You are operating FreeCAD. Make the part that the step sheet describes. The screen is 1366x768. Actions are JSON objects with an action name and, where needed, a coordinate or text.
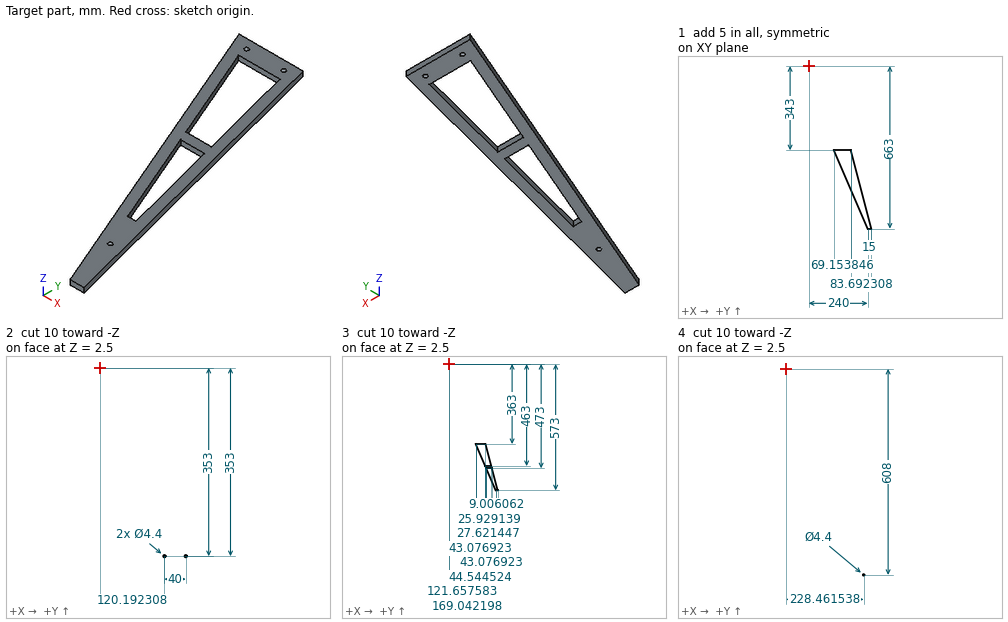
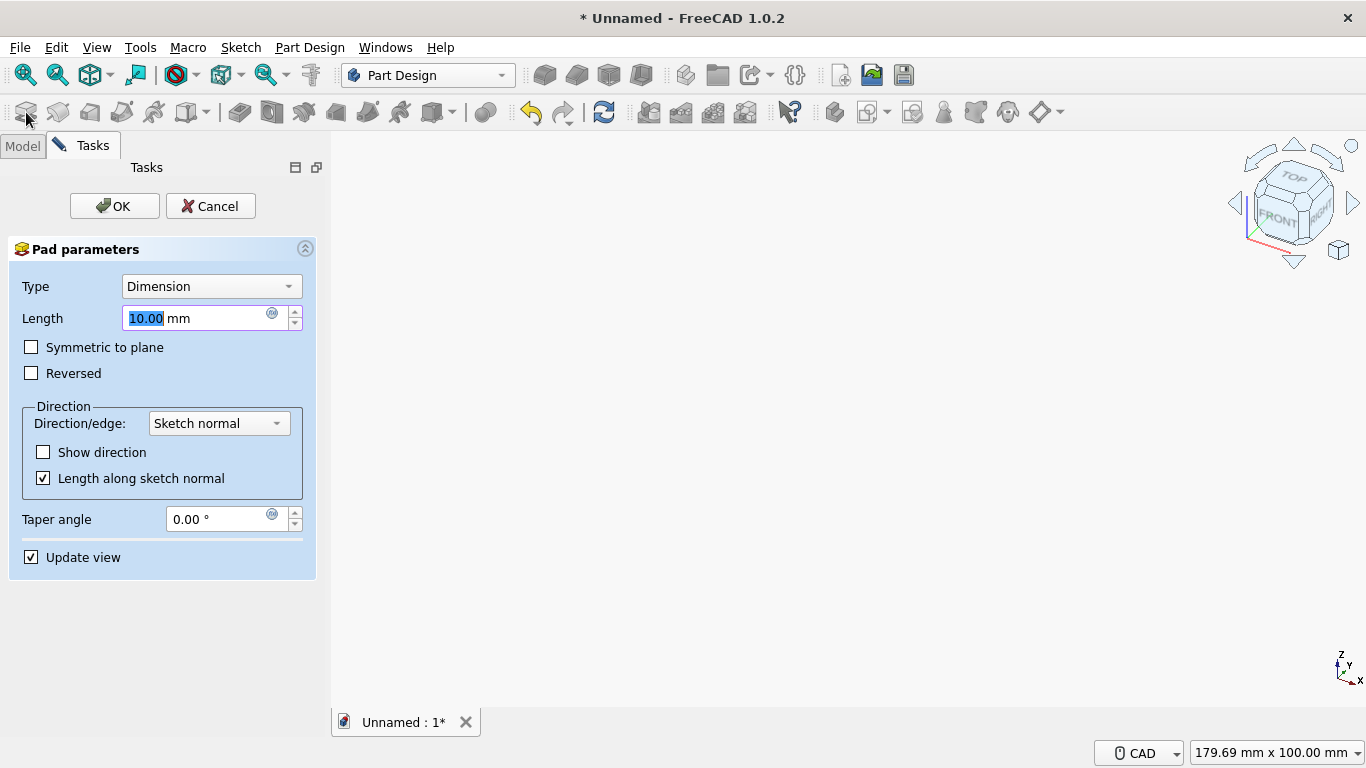
{"action": "type", "text": "5"}
{"action": "key", "text": "Tab"}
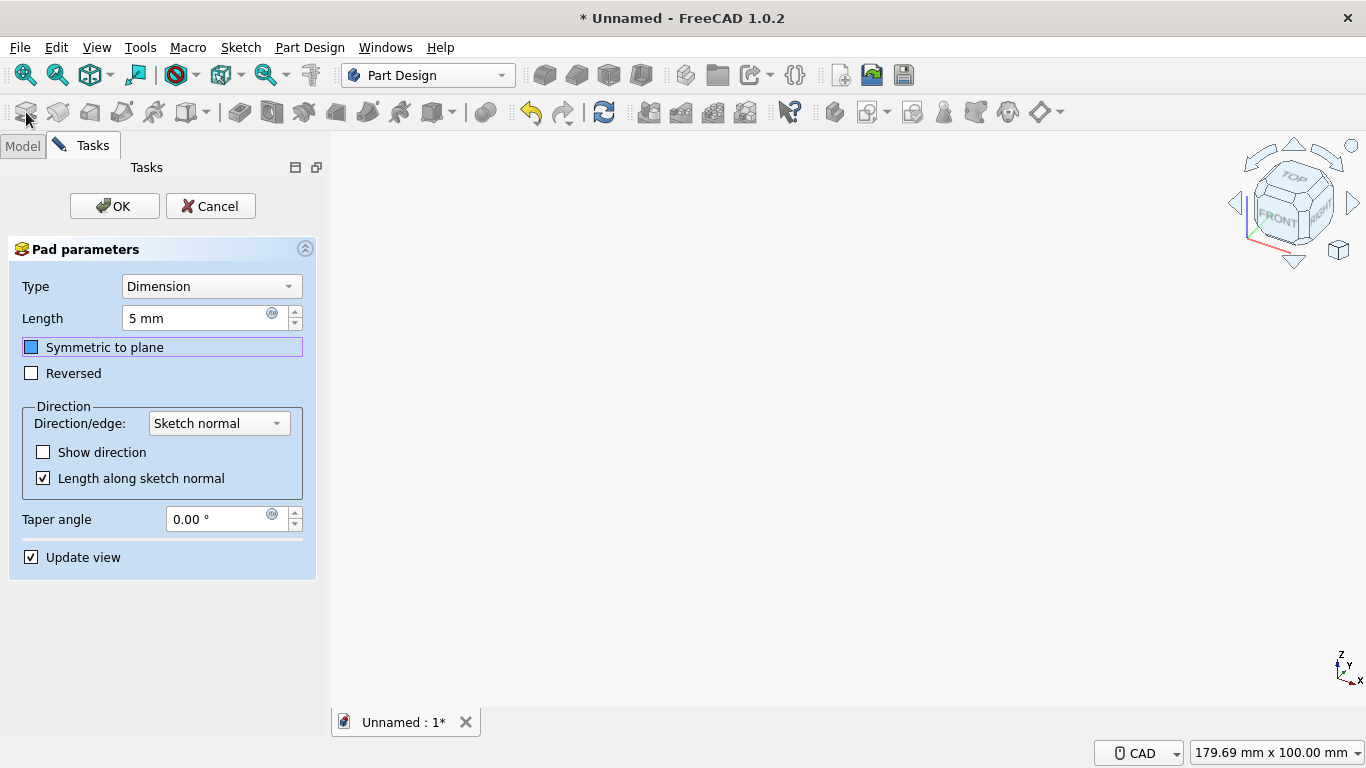
{"action": "left_click", "coordinate": [30, 347]}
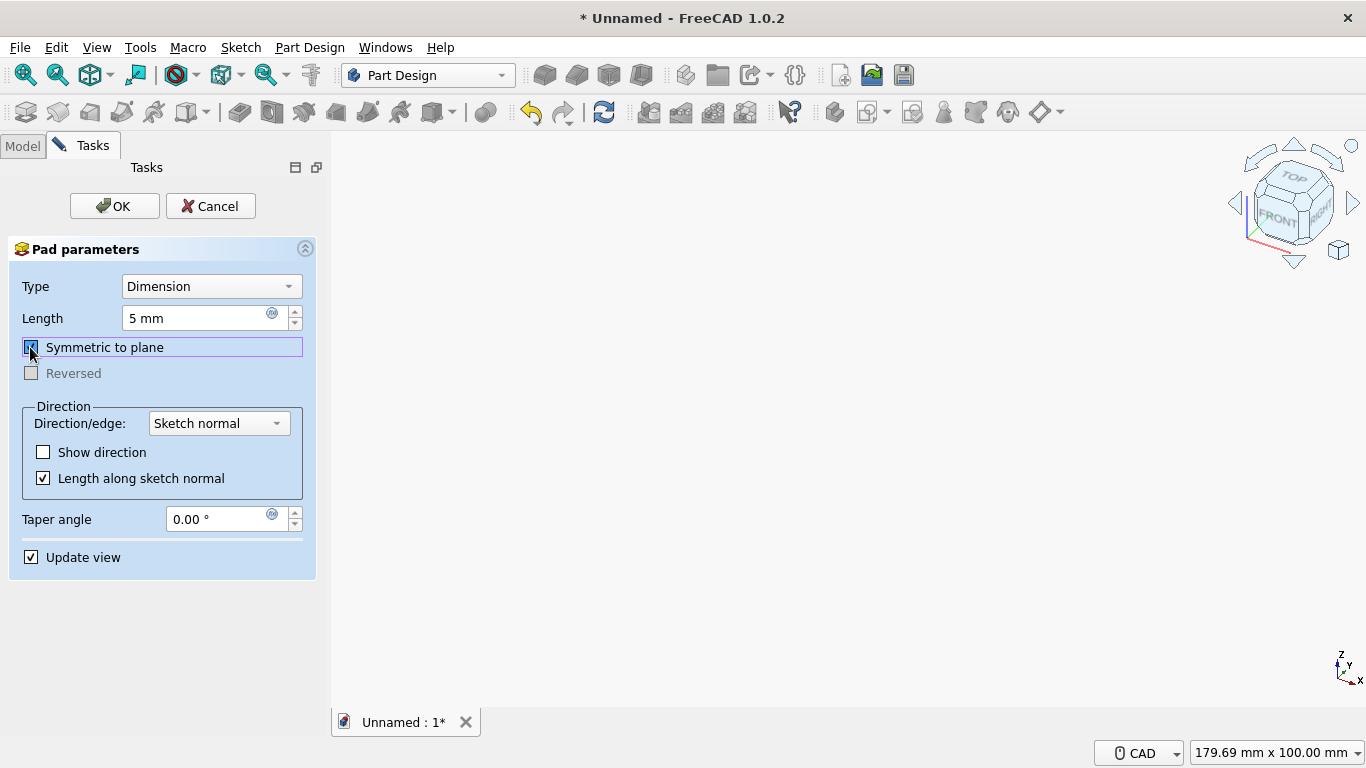
{"action": "left_click", "coordinate": [115, 206]}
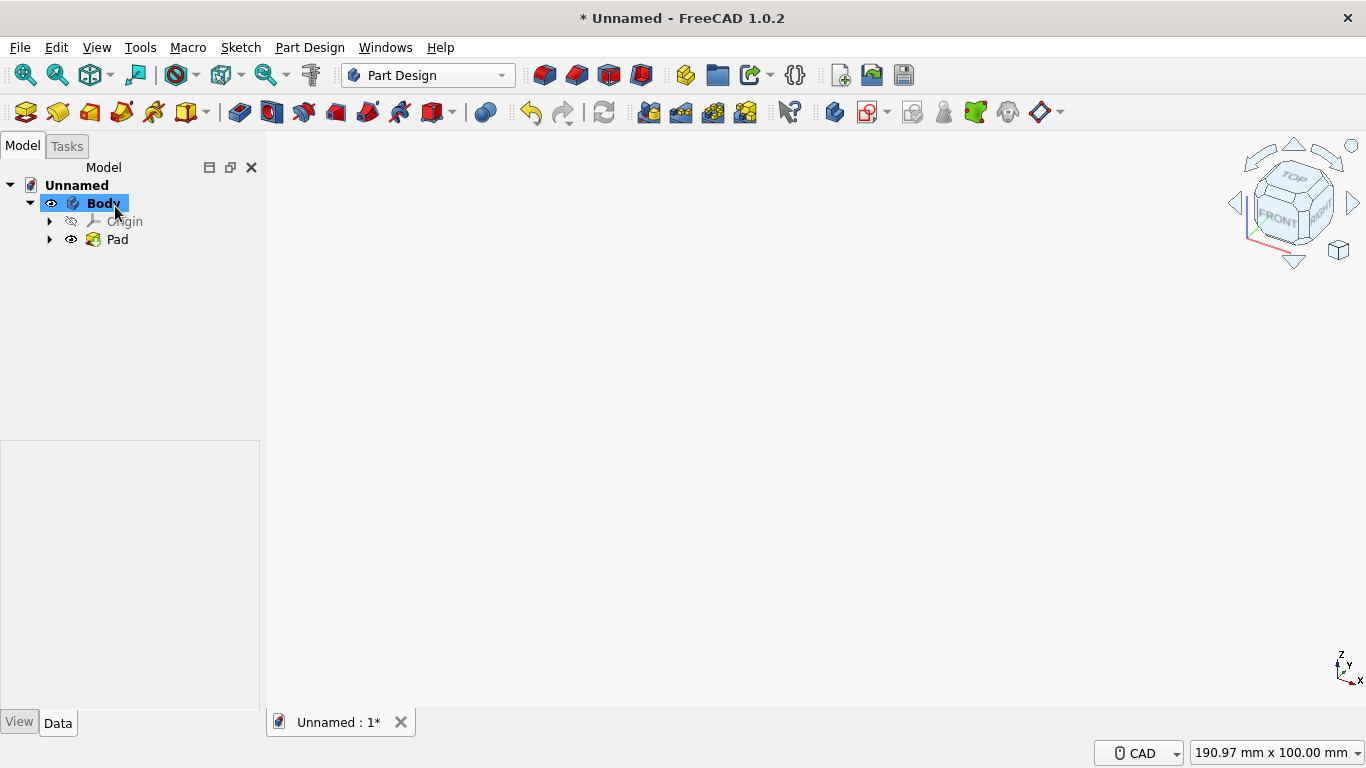
{"action": "key", "text": "v f"}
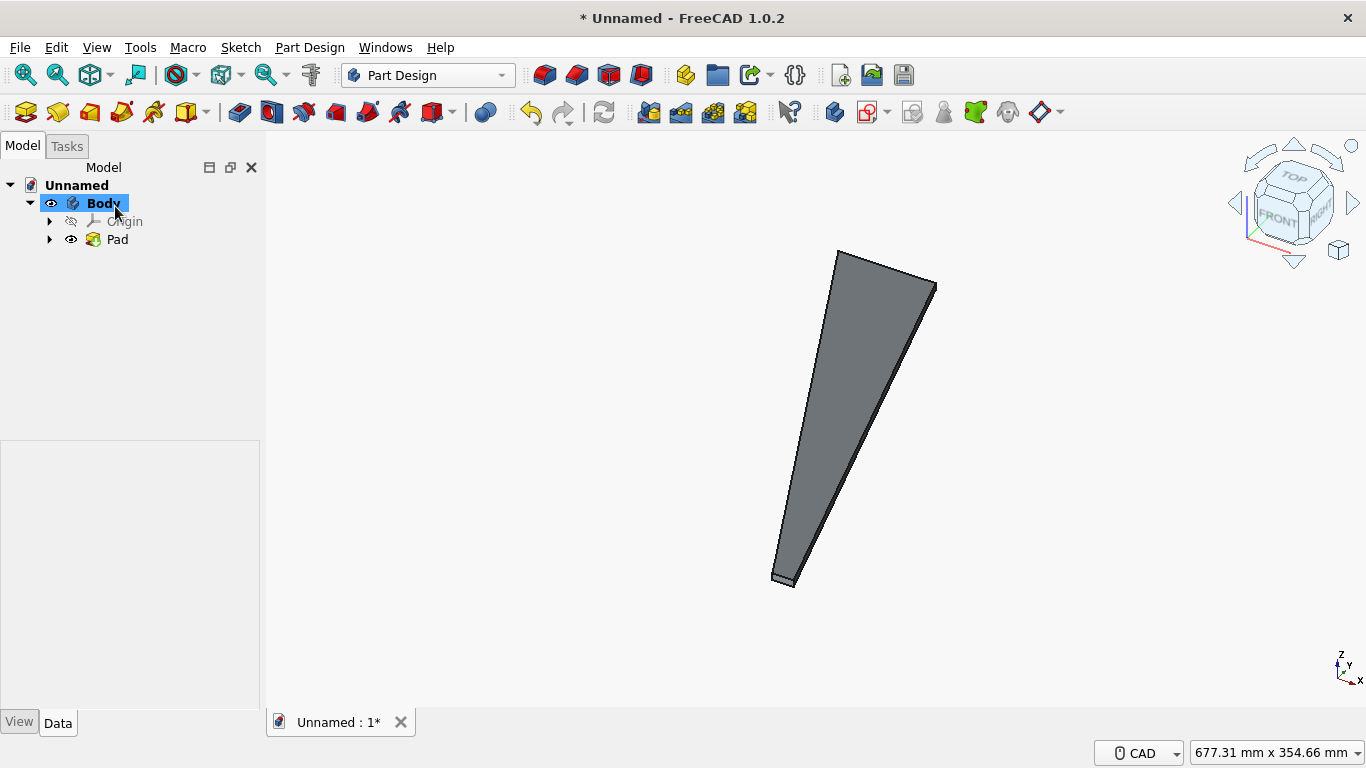
{"action": "left_click", "coordinate": [860, 331]}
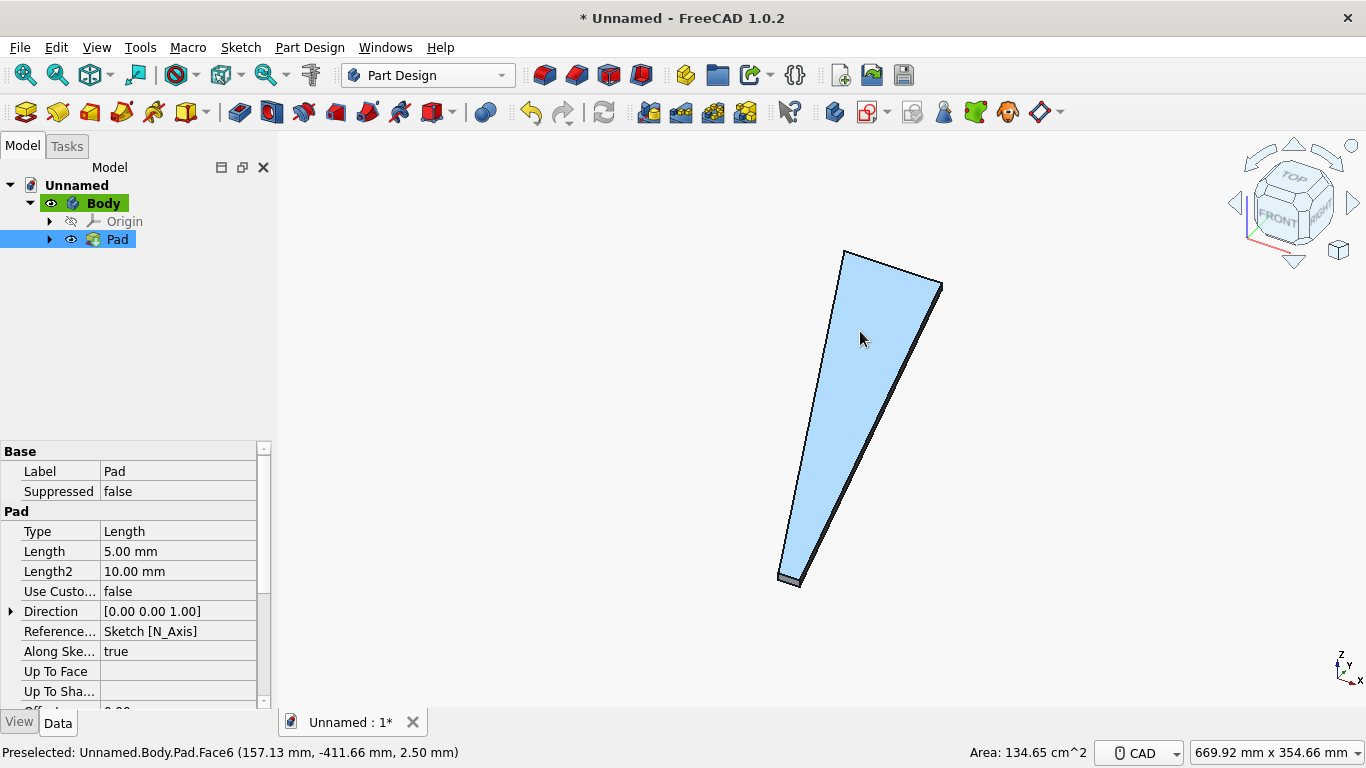
{"action": "left_click", "coordinate": [868, 112]}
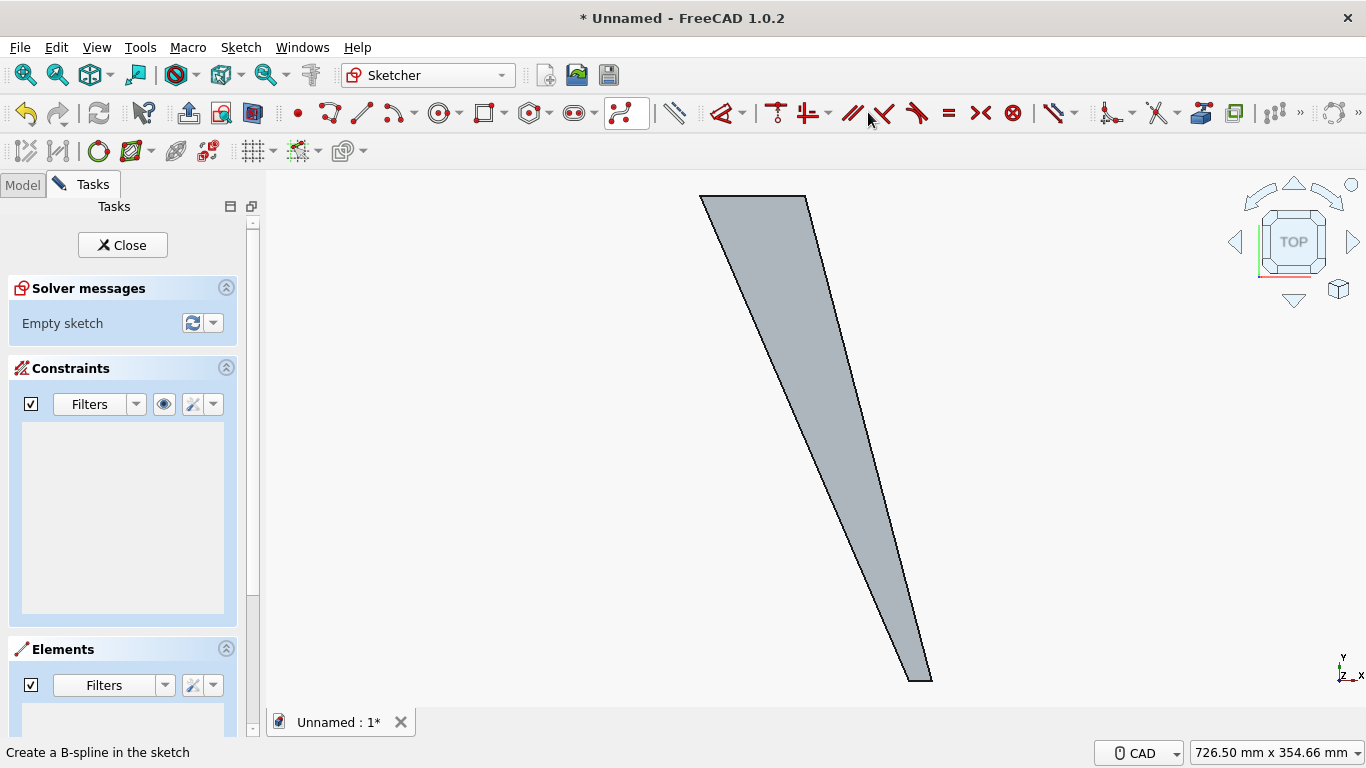
{"action": "scroll", "coordinate": [759, 198], "scroll_direction": "up", "scroll_amount": 11}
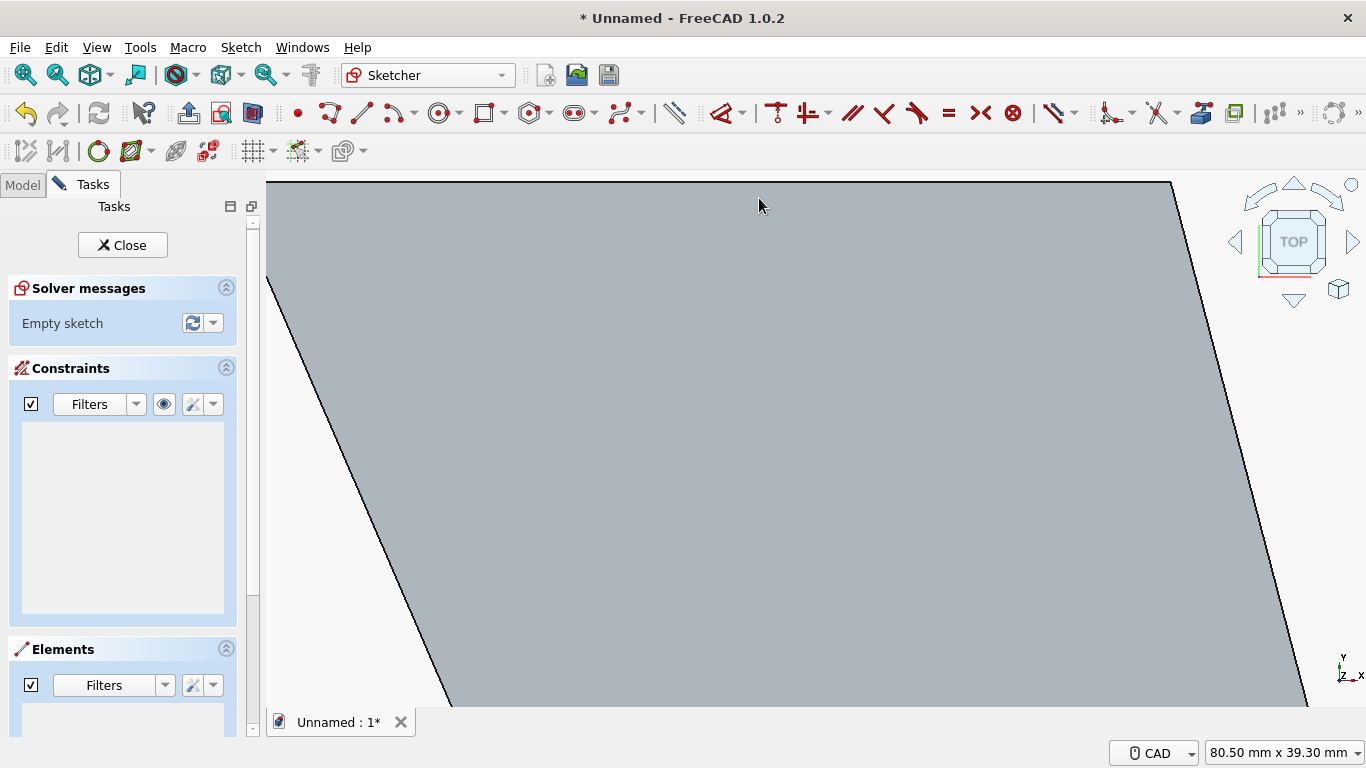
{"action": "key", "text": "g c"}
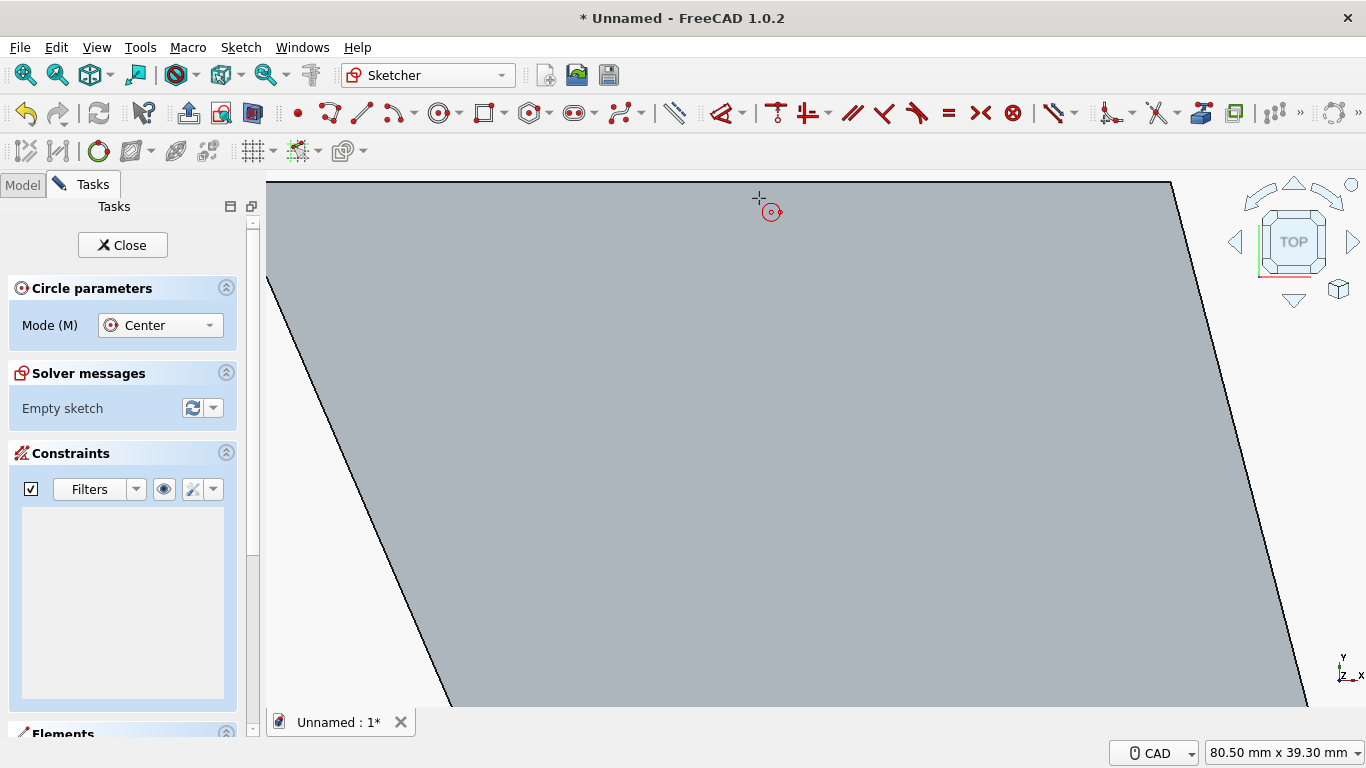
{"action": "left_click", "coordinate": [472, 318]}
{"action": "mouse_move", "coordinate": [493, 297]}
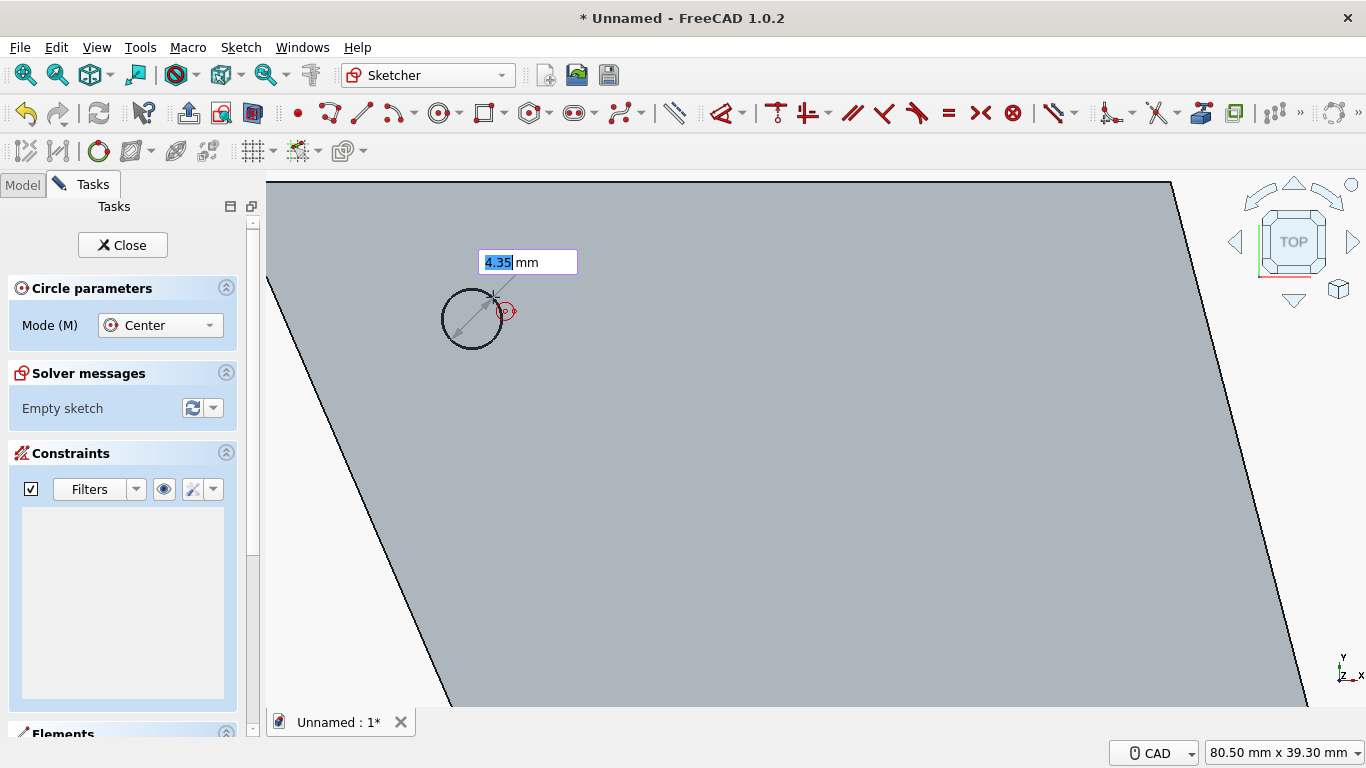
{"action": "type", "text": "4.4"}
{"action": "key", "text": "Return"}